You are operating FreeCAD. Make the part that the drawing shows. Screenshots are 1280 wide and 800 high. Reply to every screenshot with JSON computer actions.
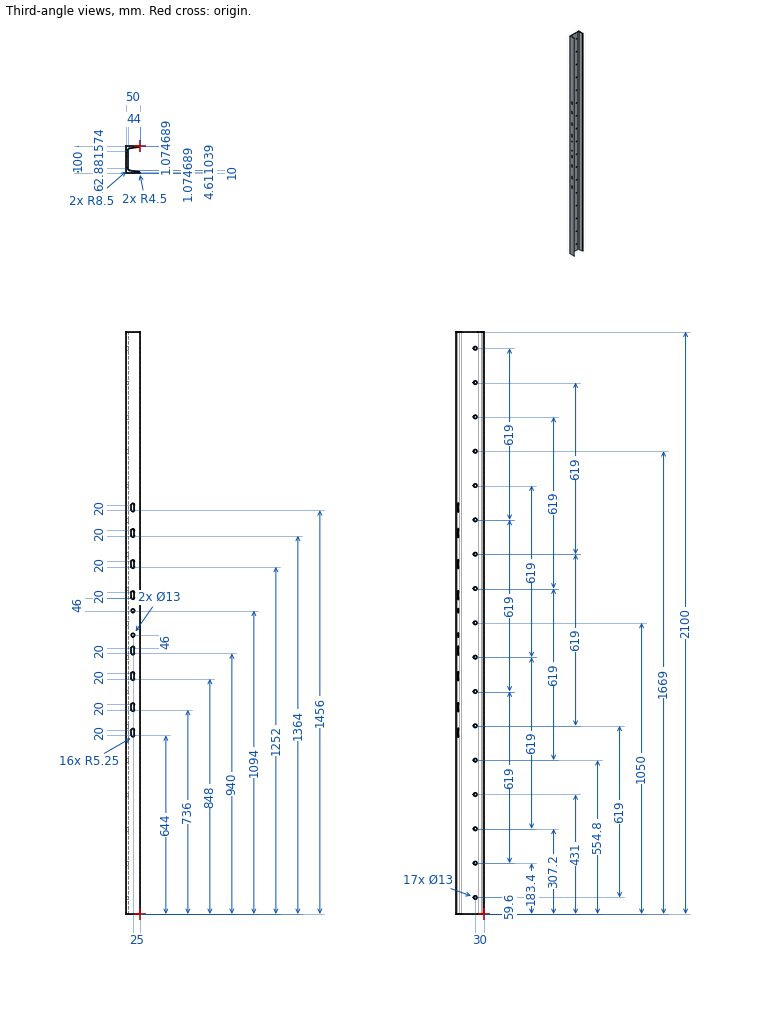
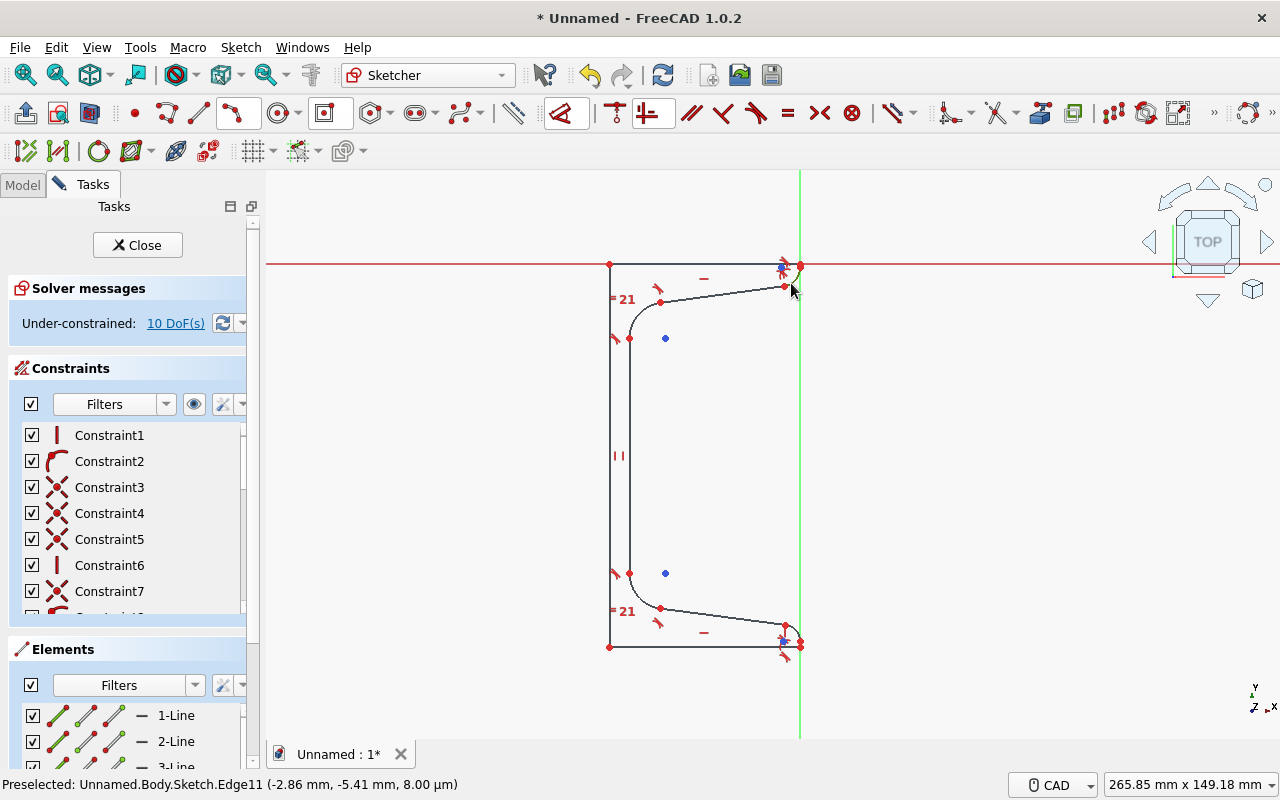
{"action": "scroll", "coordinate": [799, 634], "scroll_direction": "up", "scroll_amount": 4}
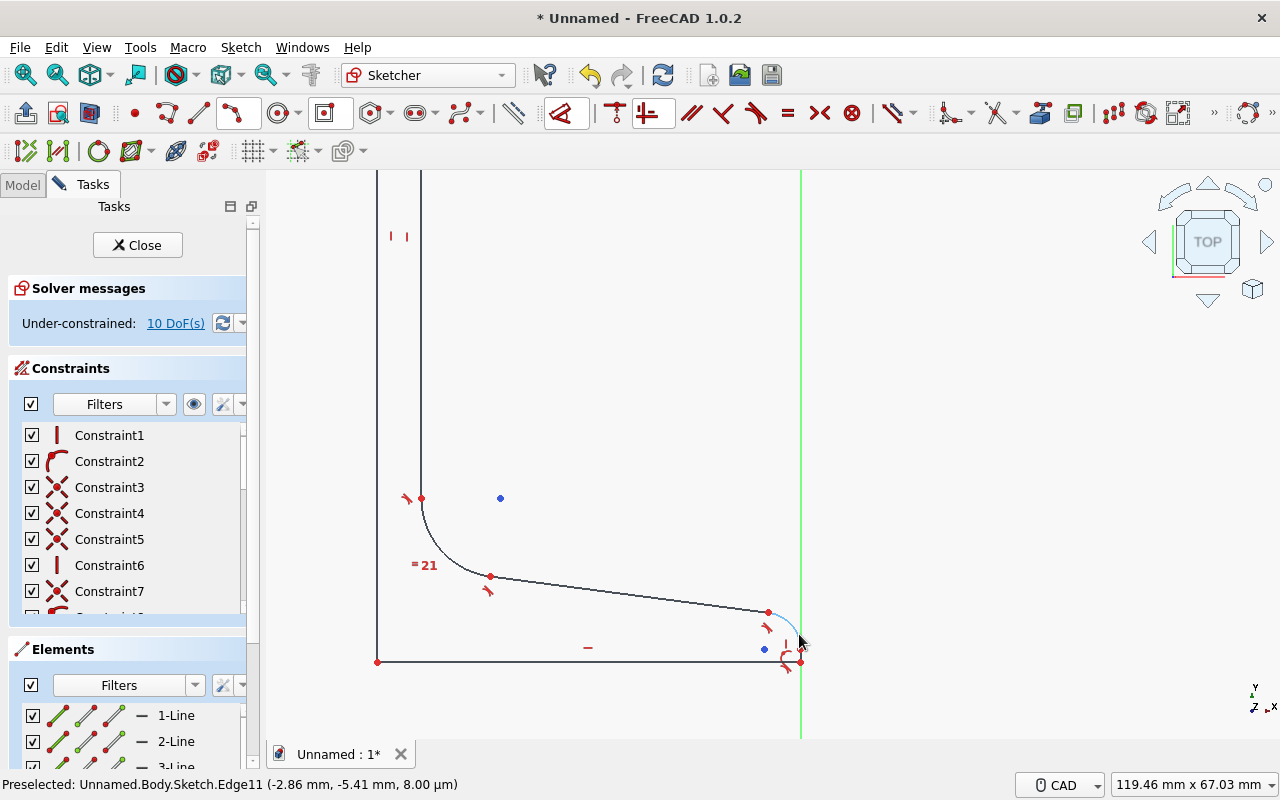
{"action": "left_click", "coordinate": [797, 634]}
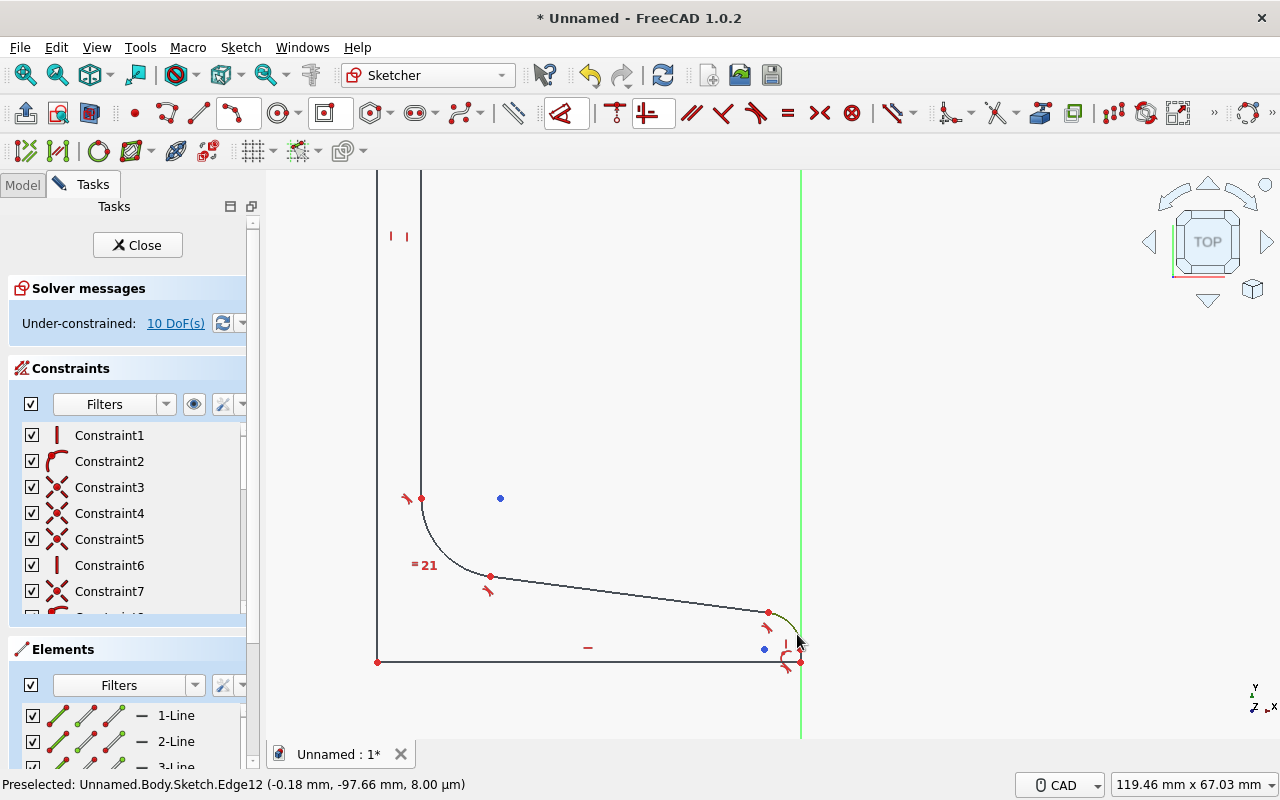
{"action": "left_click", "coordinate": [788, 114]}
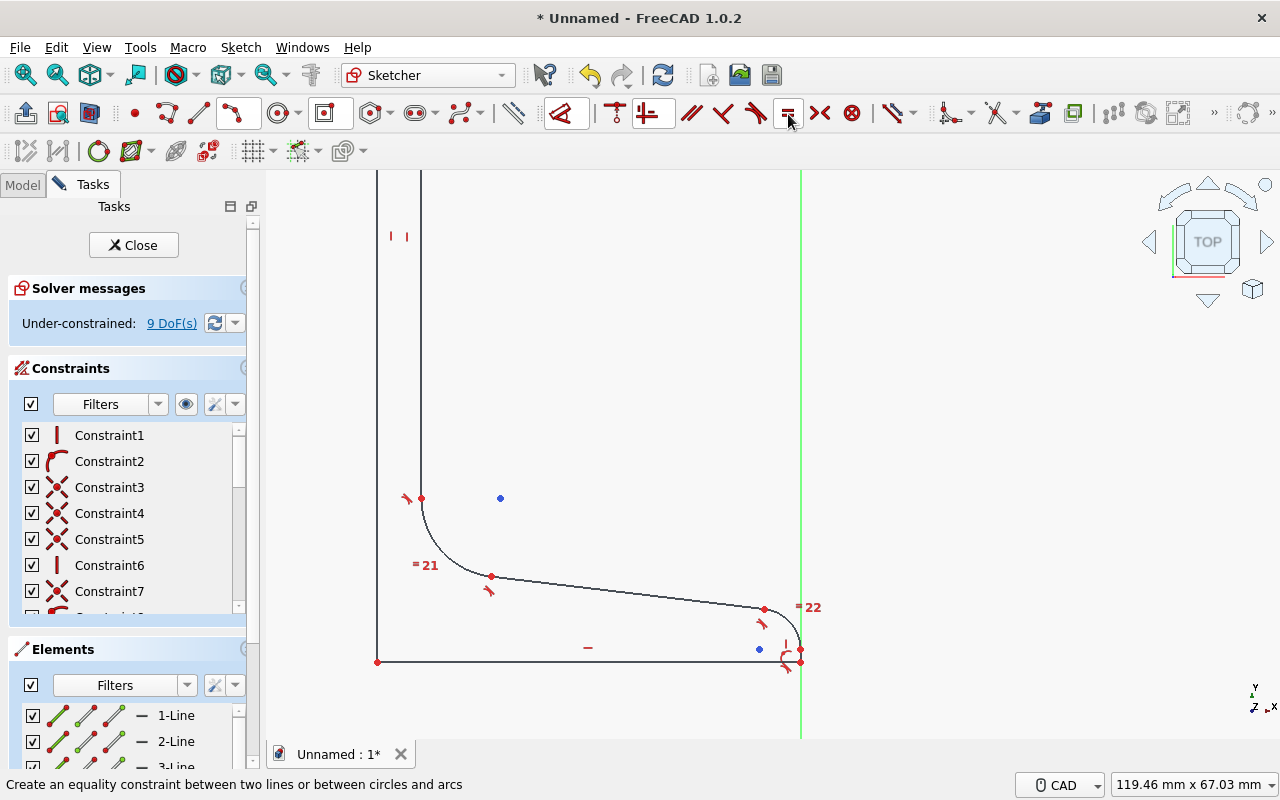
{"action": "key", "text": "d"}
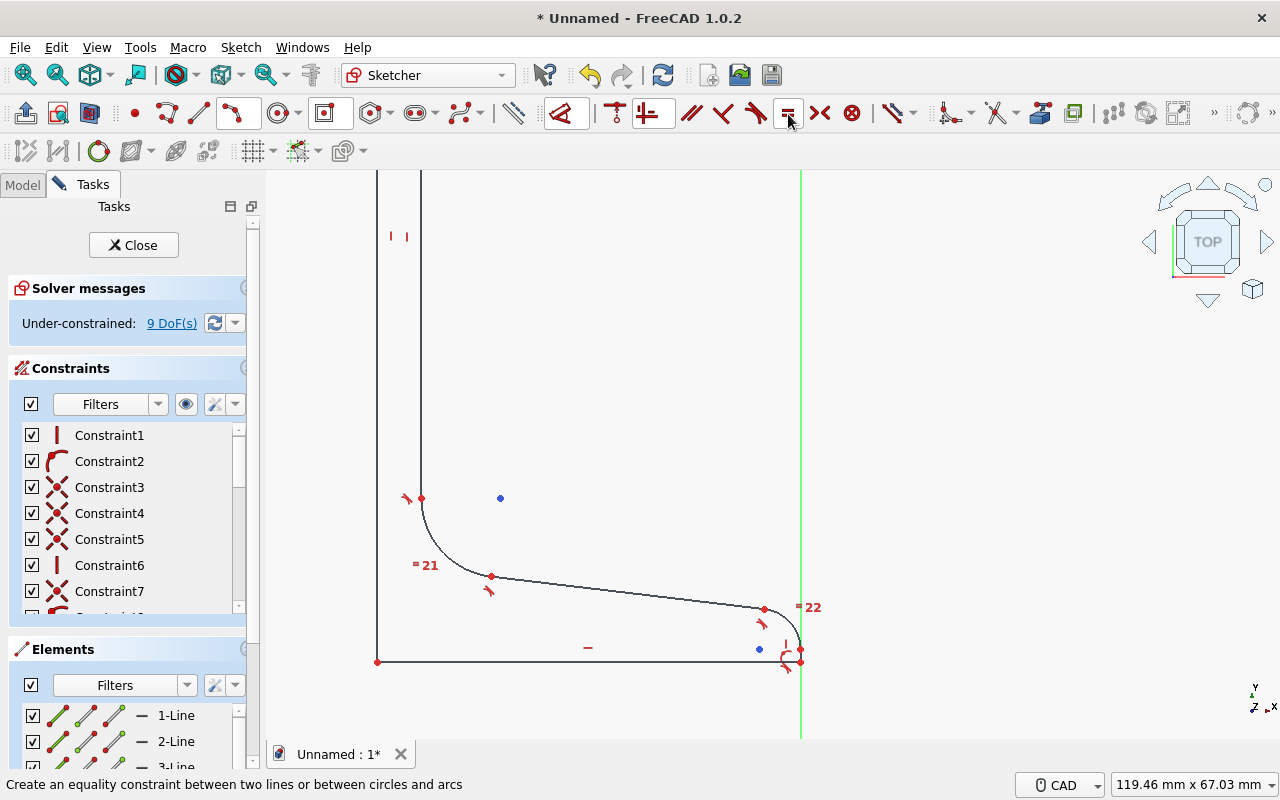
{"action": "left_click", "coordinate": [429, 532]}
{"action": "left_click", "coordinate": [400, 546]}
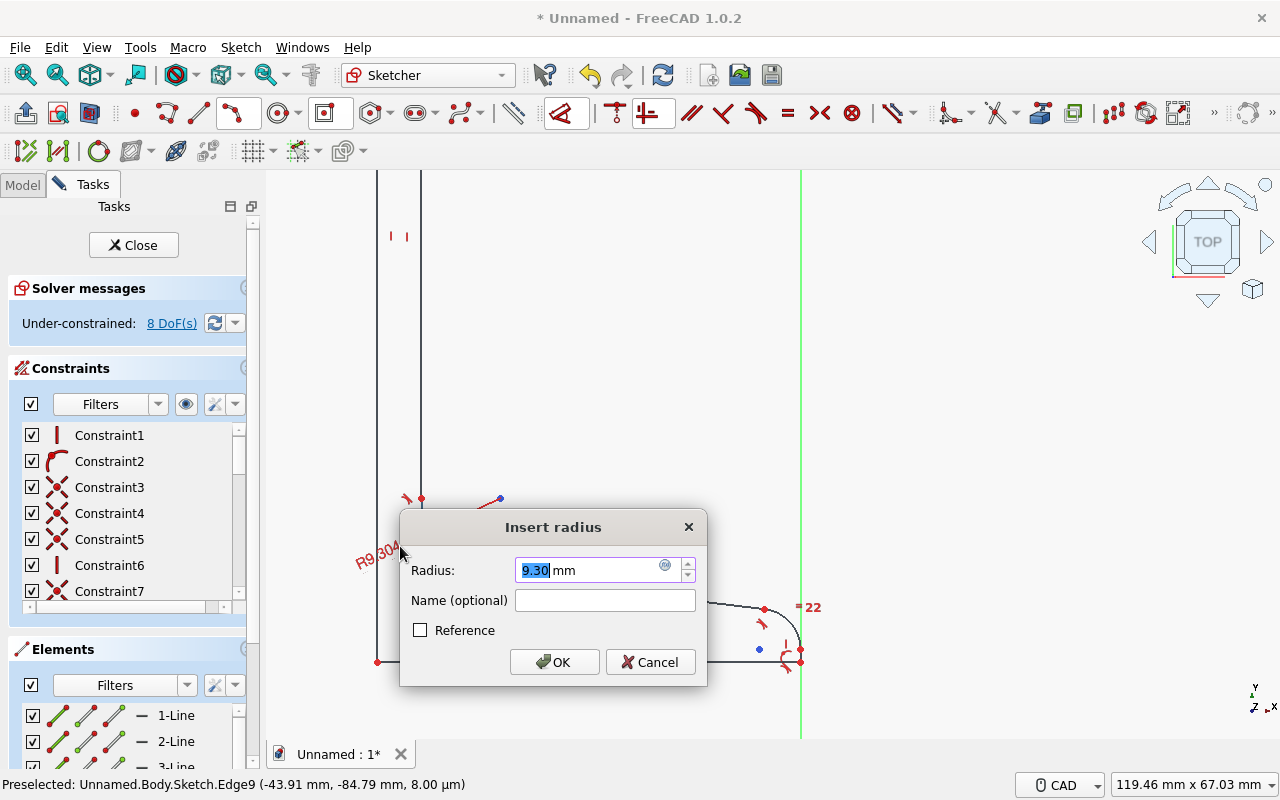
{"action": "type", "text": "8.5"}
{"action": "key", "text": "Return"}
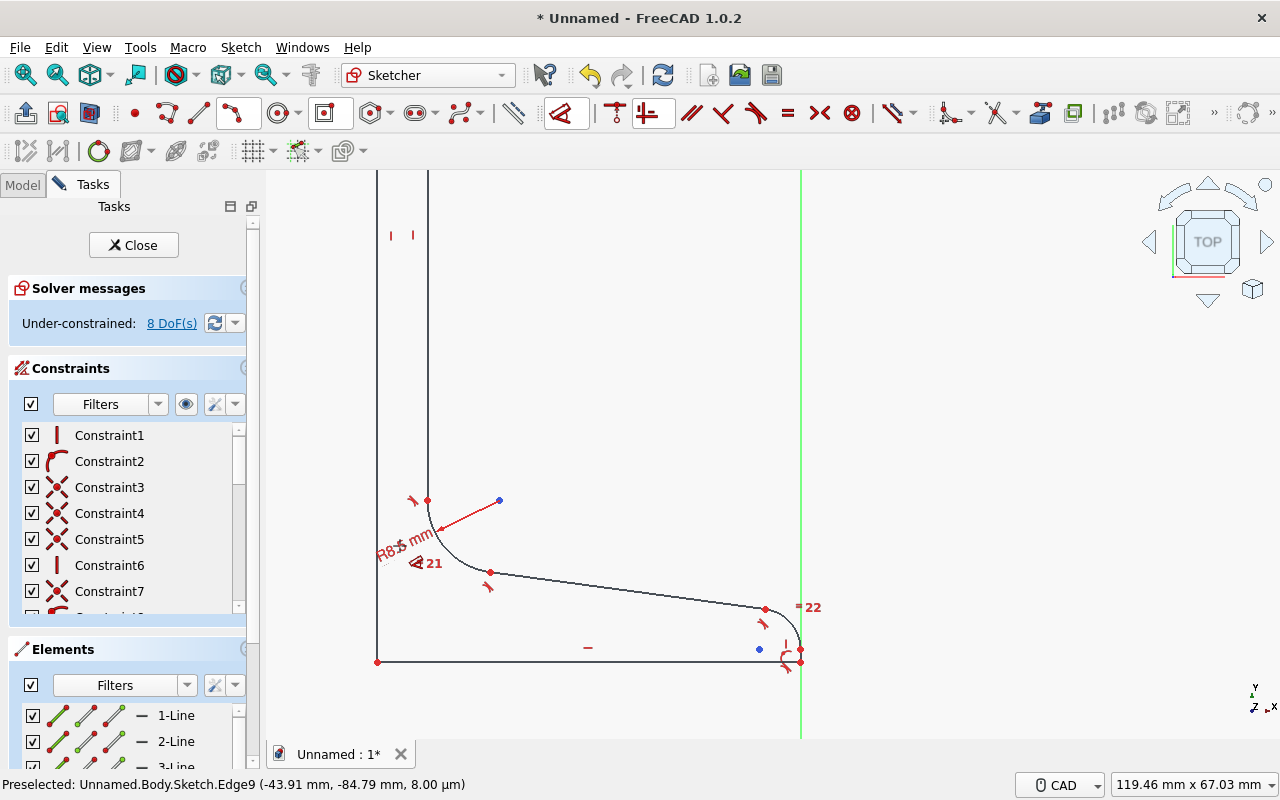
{"action": "scroll", "coordinate": [799, 634], "scroll_direction": "down", "scroll_amount": 4}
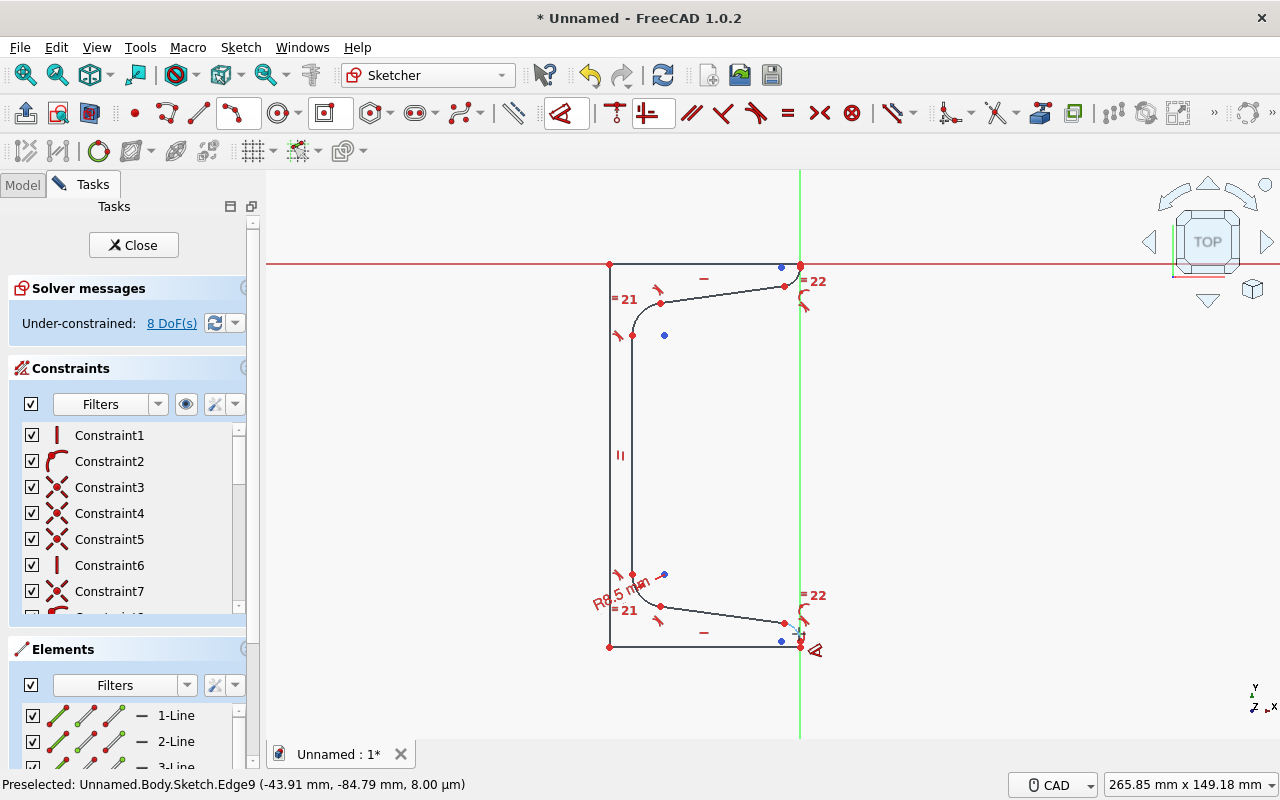
{"action": "scroll", "coordinate": [791, 283], "scroll_direction": "up", "scroll_amount": 5}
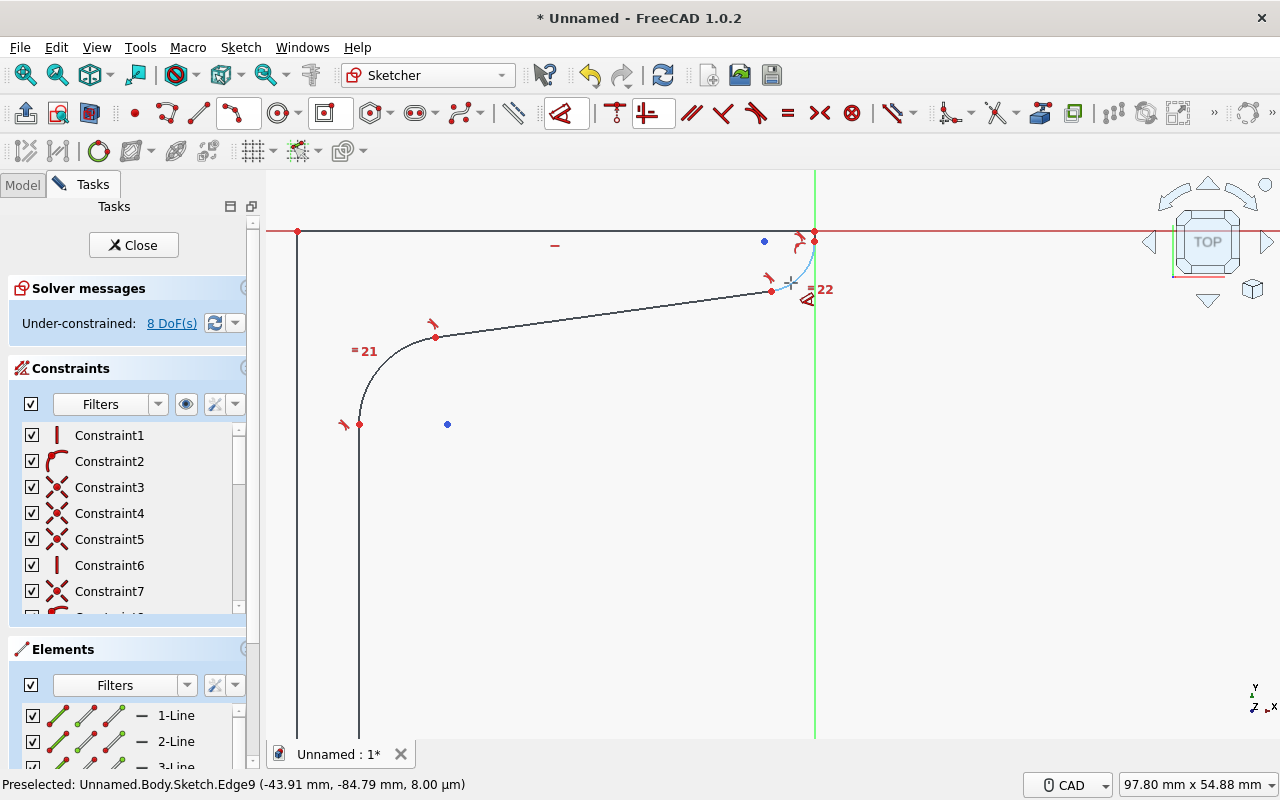
{"action": "left_click", "coordinate": [791, 284]}
{"action": "left_click", "coordinate": [769, 323]}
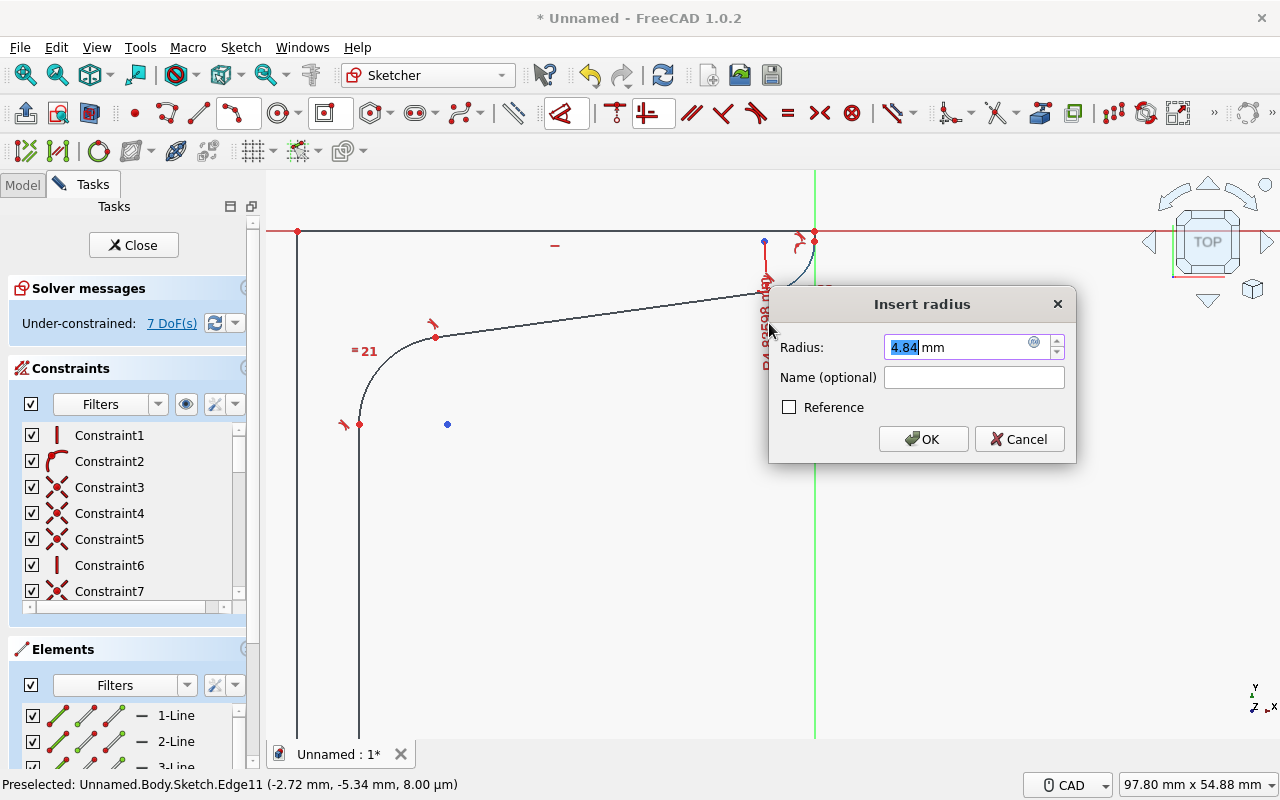
{"action": "type", "text": "4.5"}
{"action": "key", "text": "Return"}